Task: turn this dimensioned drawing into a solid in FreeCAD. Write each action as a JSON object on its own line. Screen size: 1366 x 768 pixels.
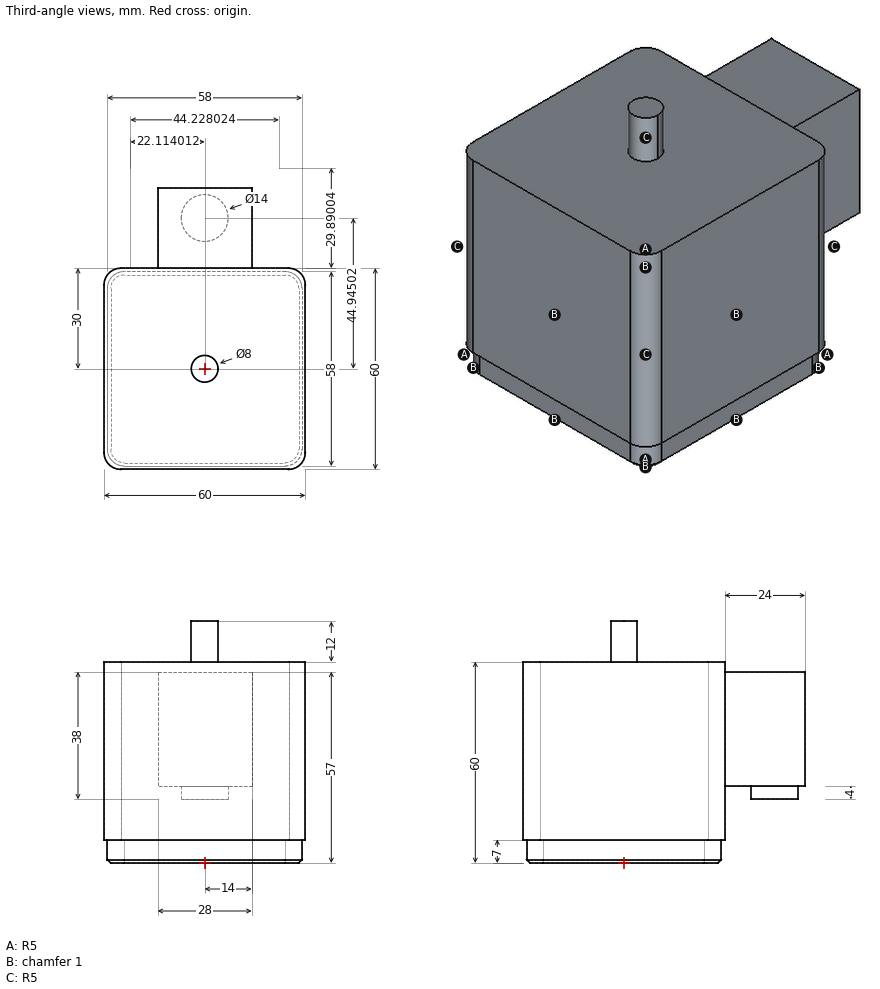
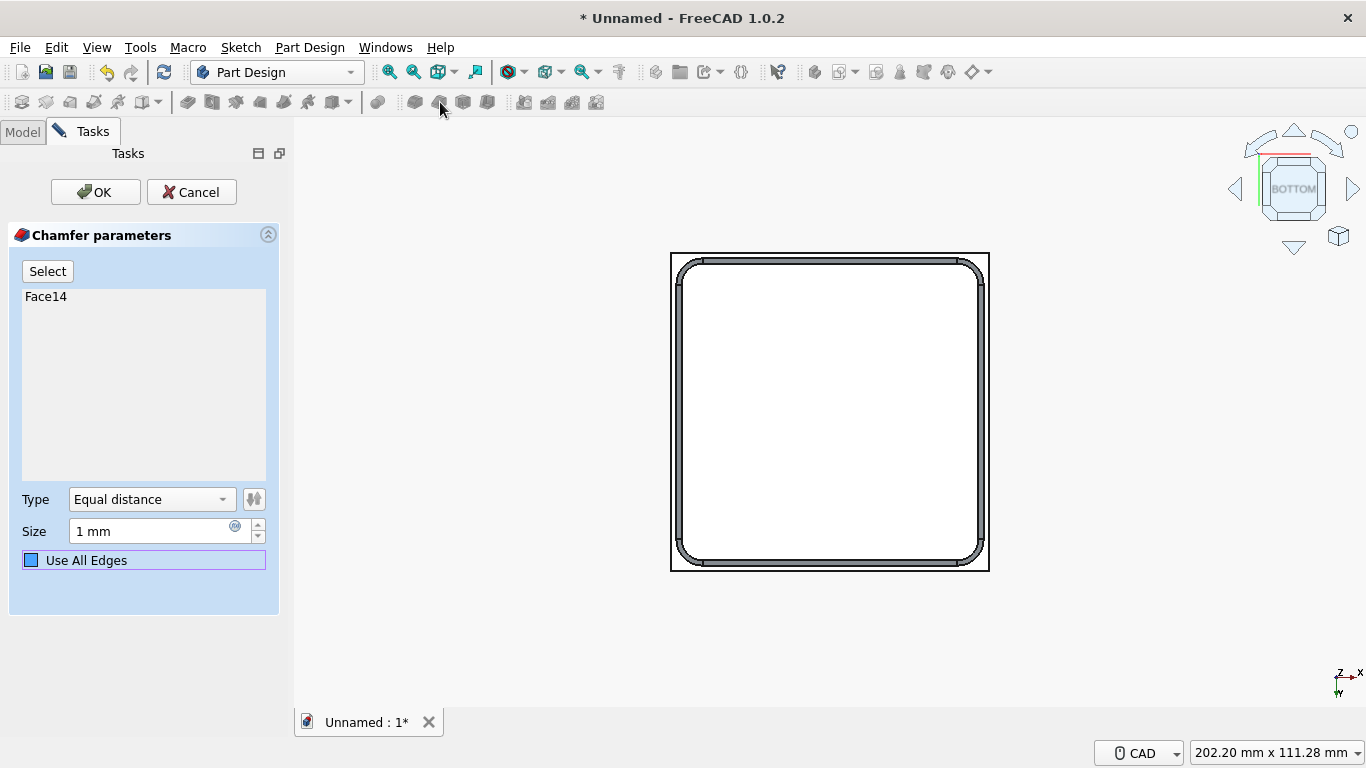
{"action": "left_click", "coordinate": [96, 192]}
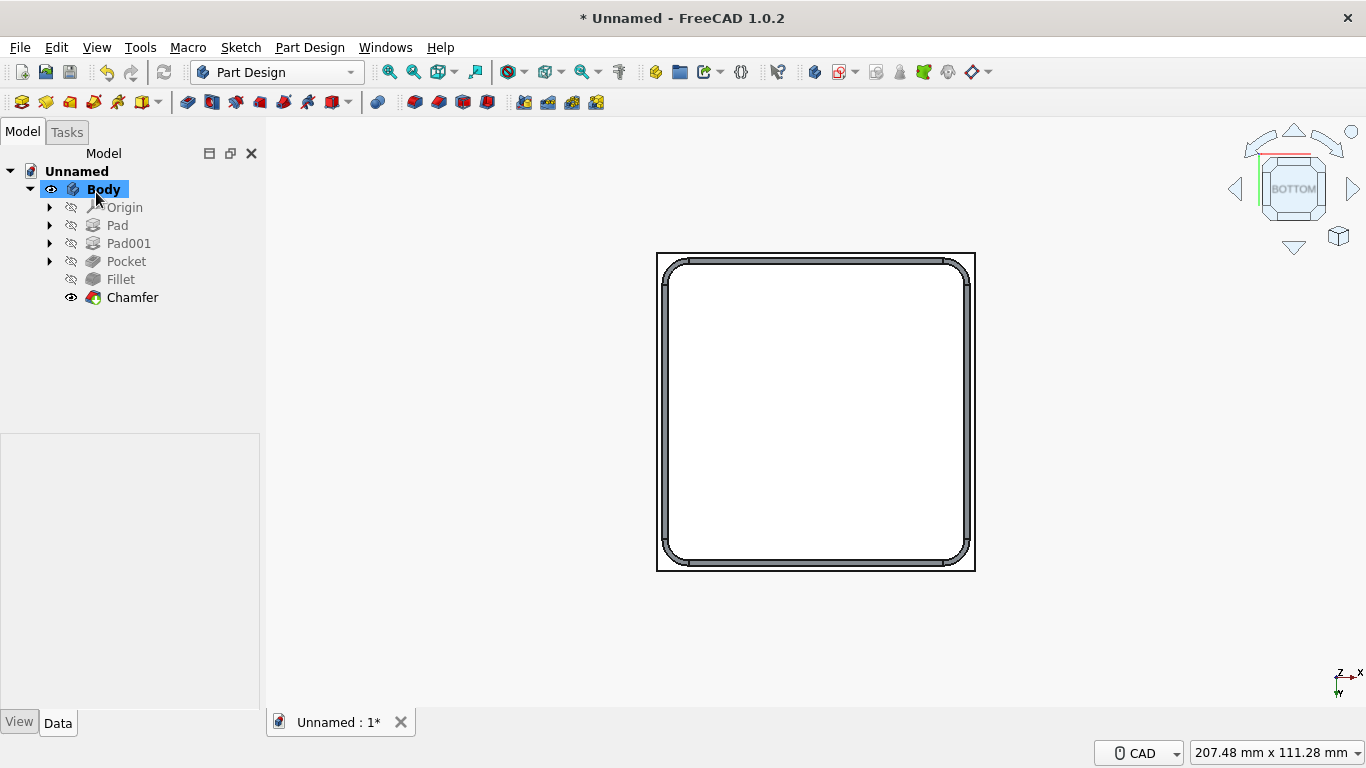
{"action": "key", "text": "0"}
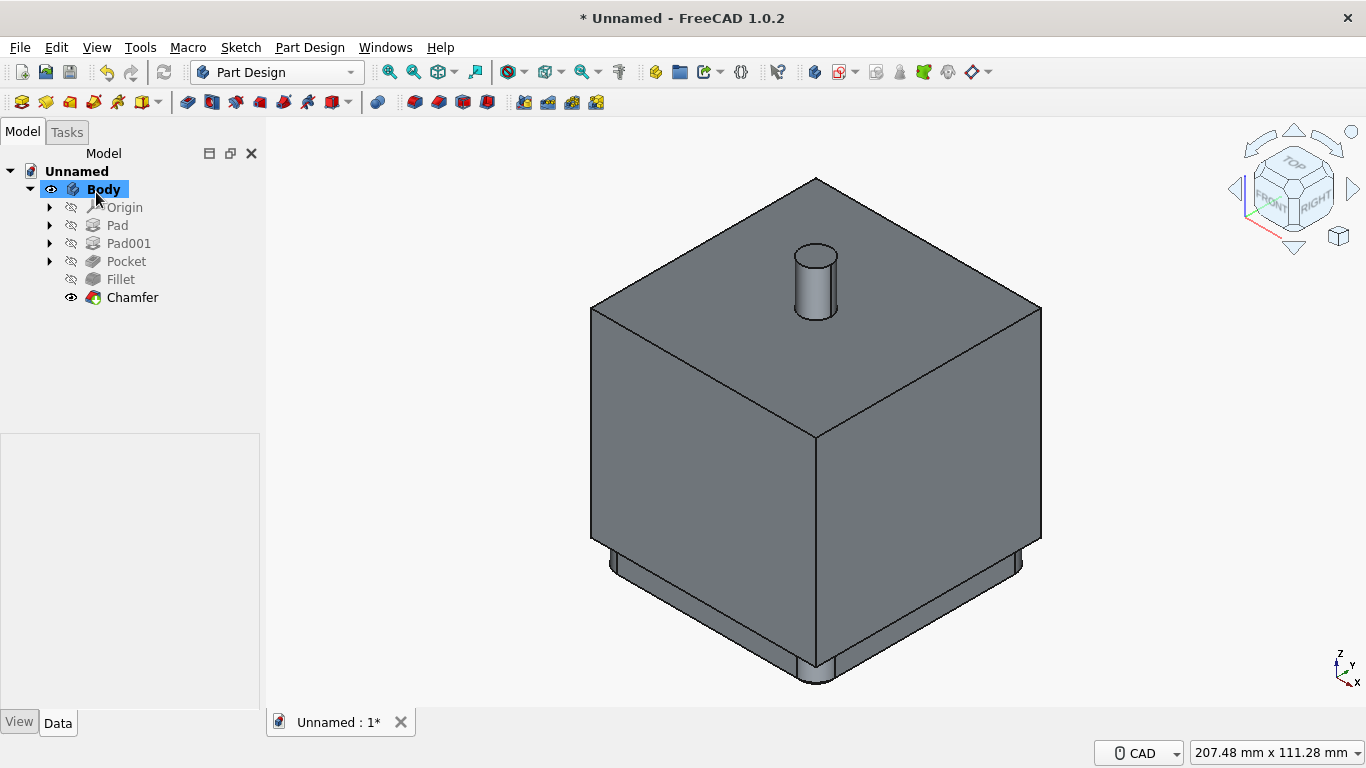
{"action": "left_click", "coordinate": [816, 552]}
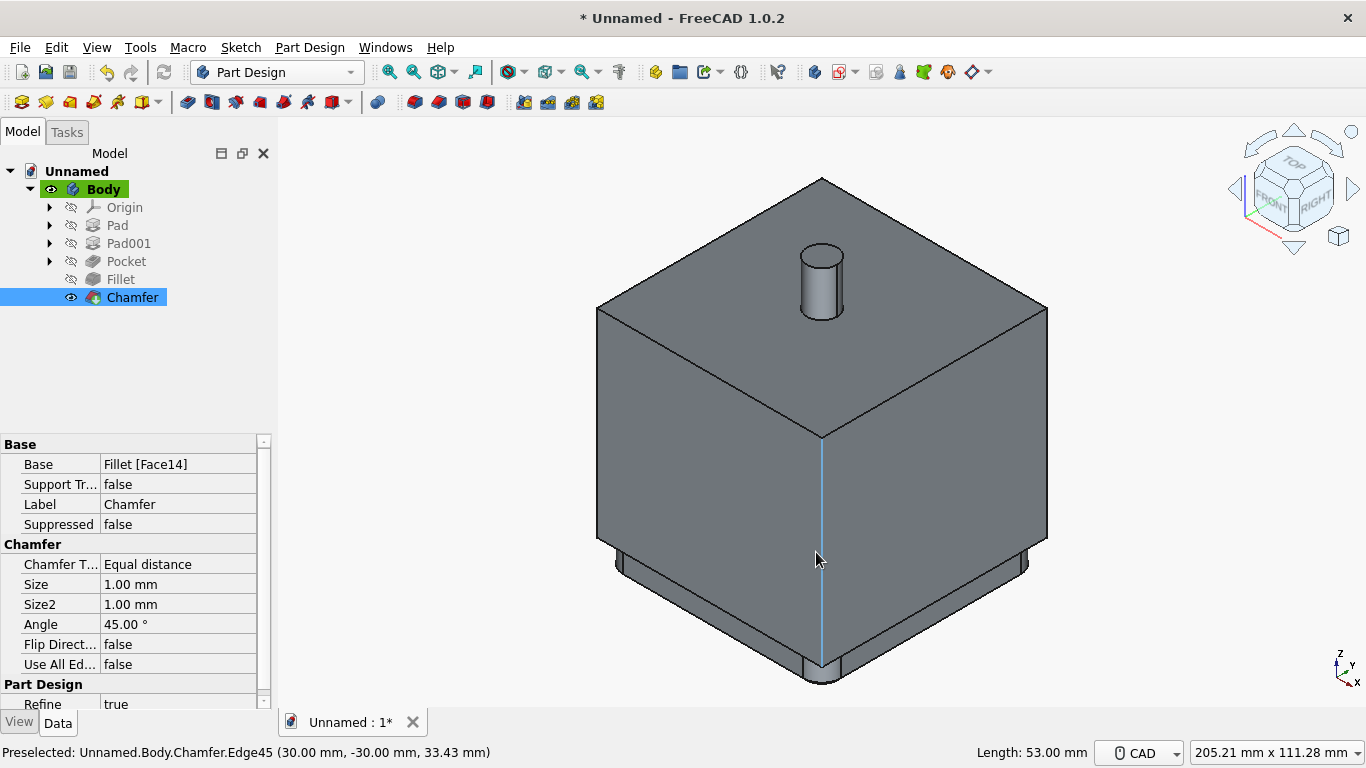
{"action": "key", "text": "2"}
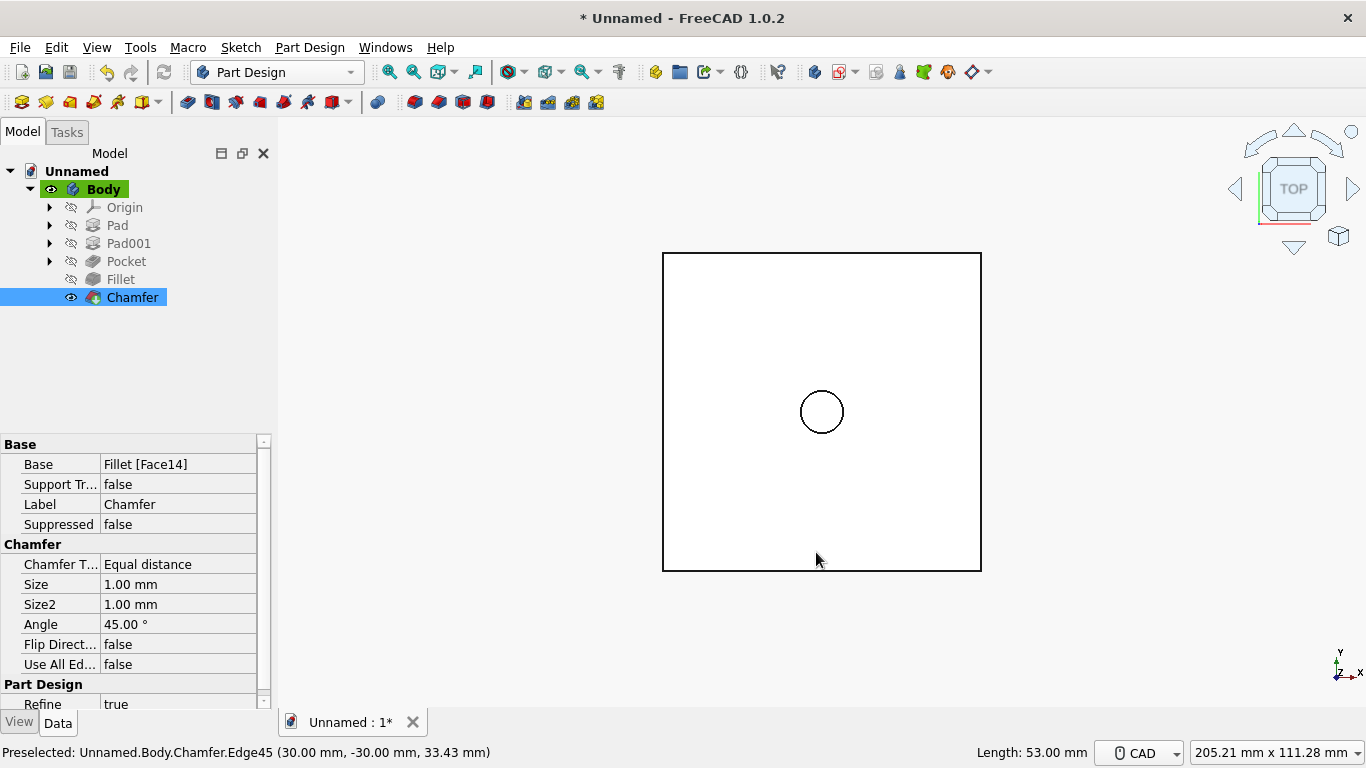
{"action": "key", "text": "1"}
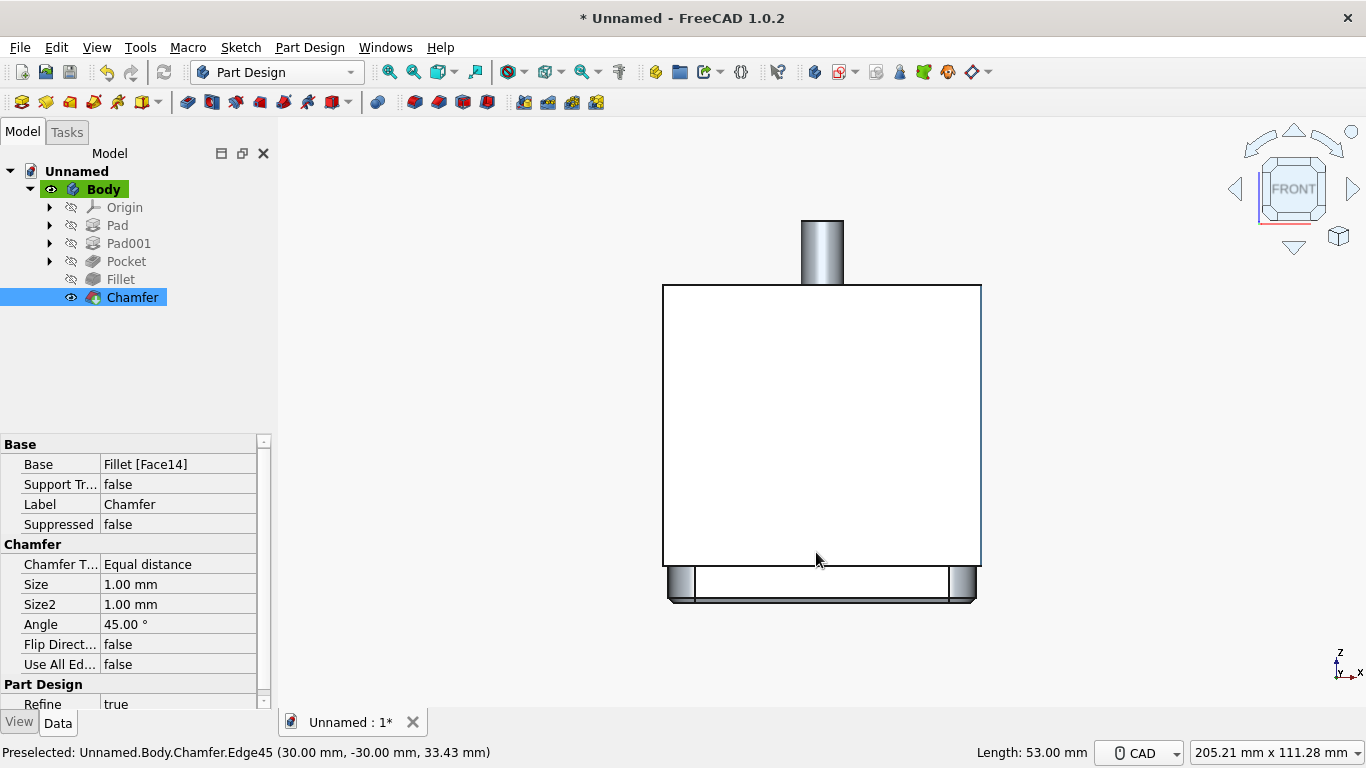
{"action": "left_click", "coordinate": [663, 424], "text": "ctrl"}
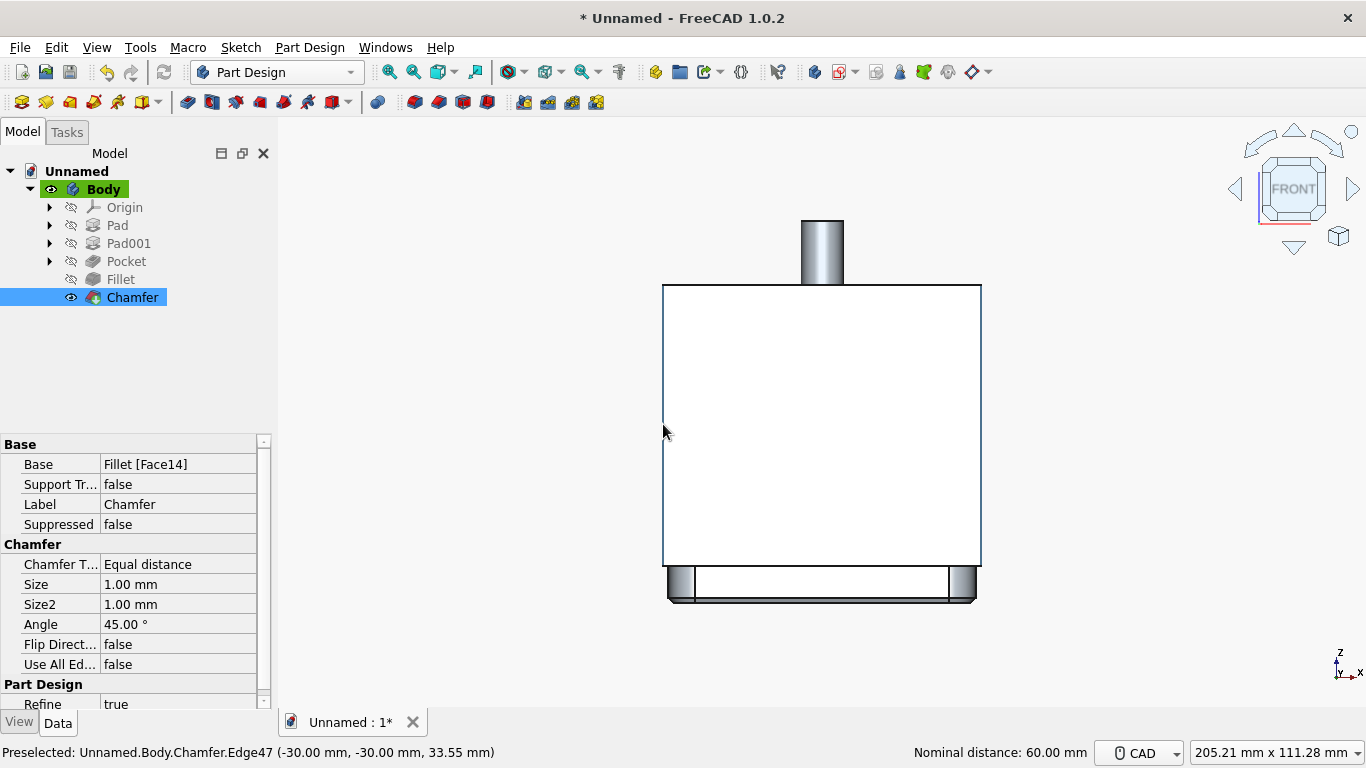
{"action": "key", "text": "3"}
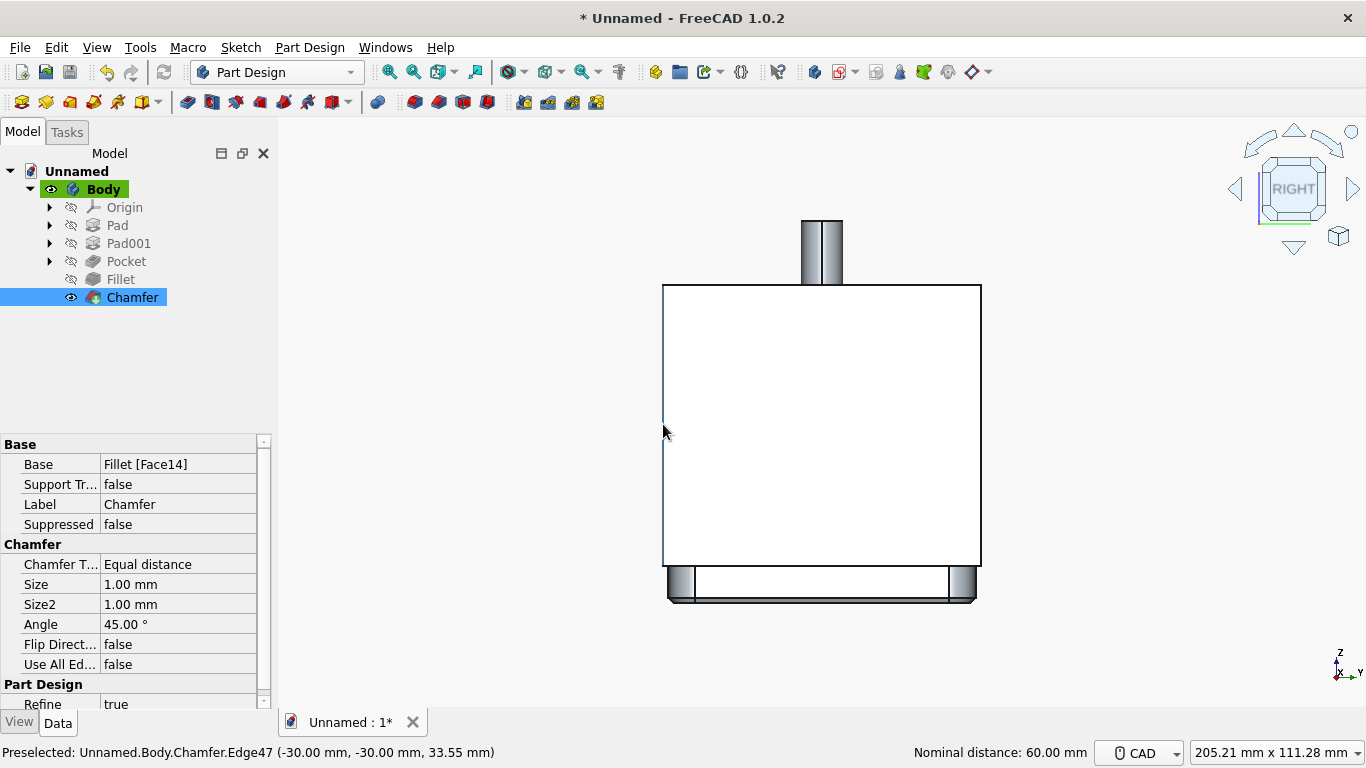
{"action": "left_click", "coordinate": [981, 424], "text": "ctrl"}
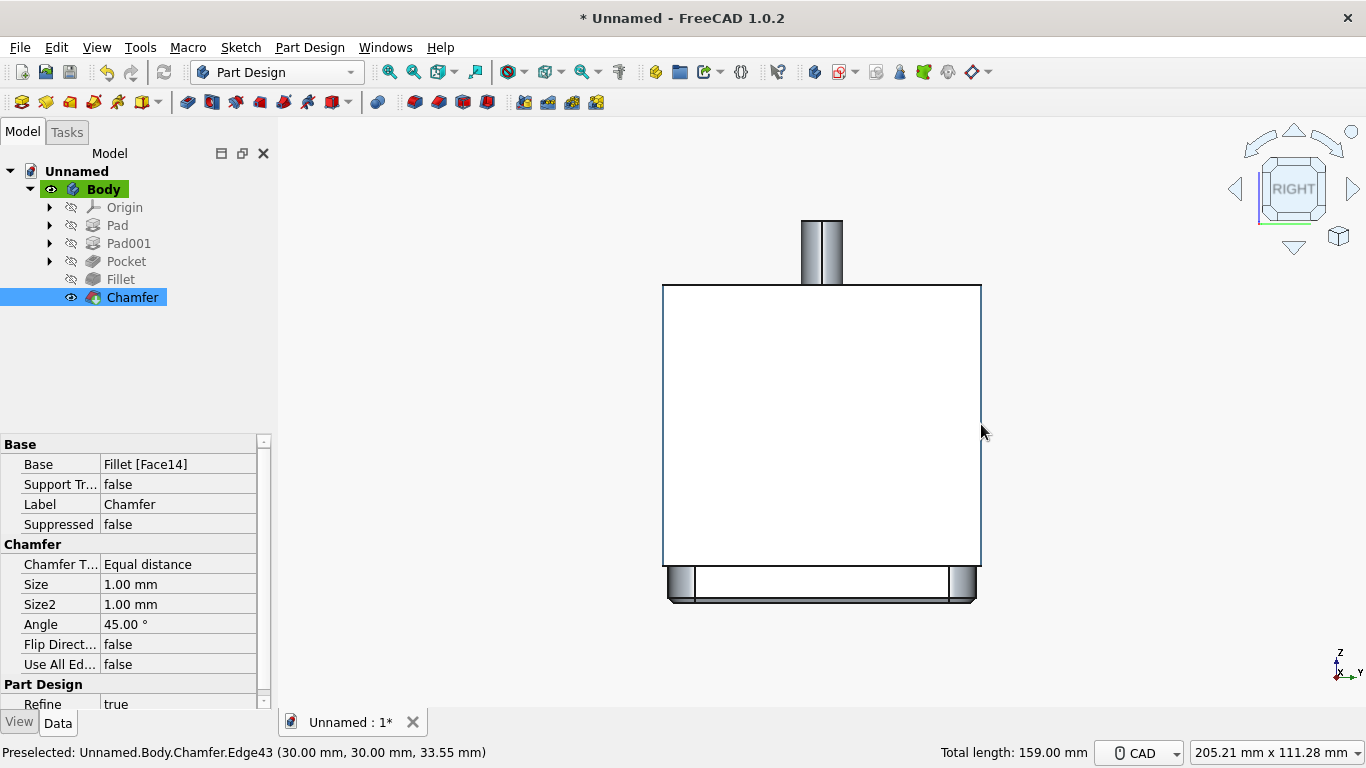
{"action": "key", "text": "5"}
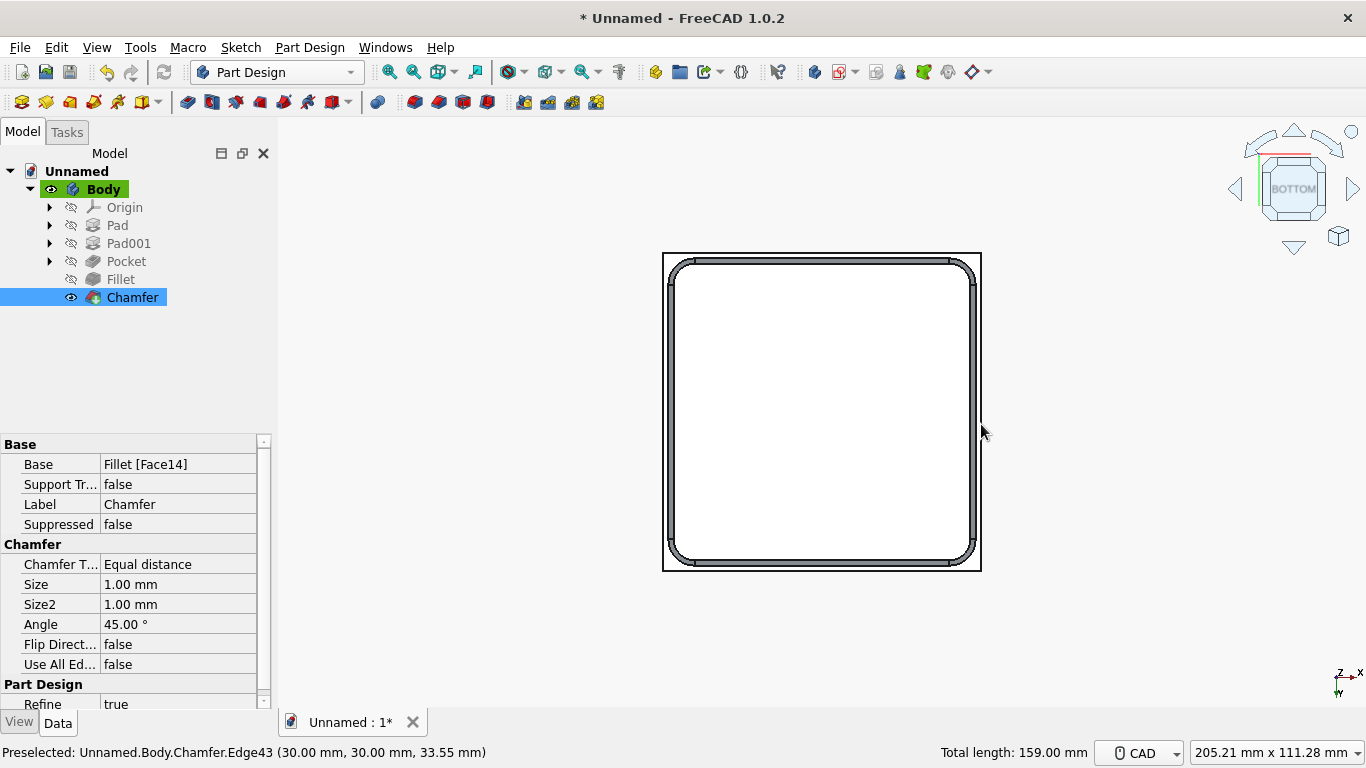
{"action": "key", "text": "4"}